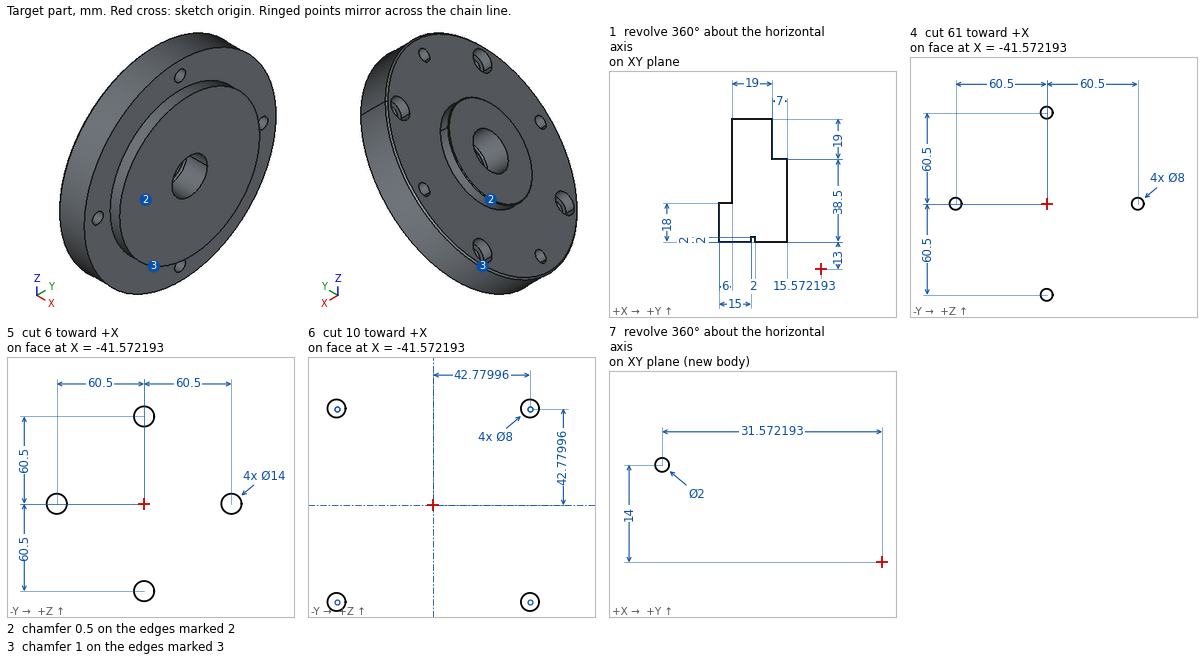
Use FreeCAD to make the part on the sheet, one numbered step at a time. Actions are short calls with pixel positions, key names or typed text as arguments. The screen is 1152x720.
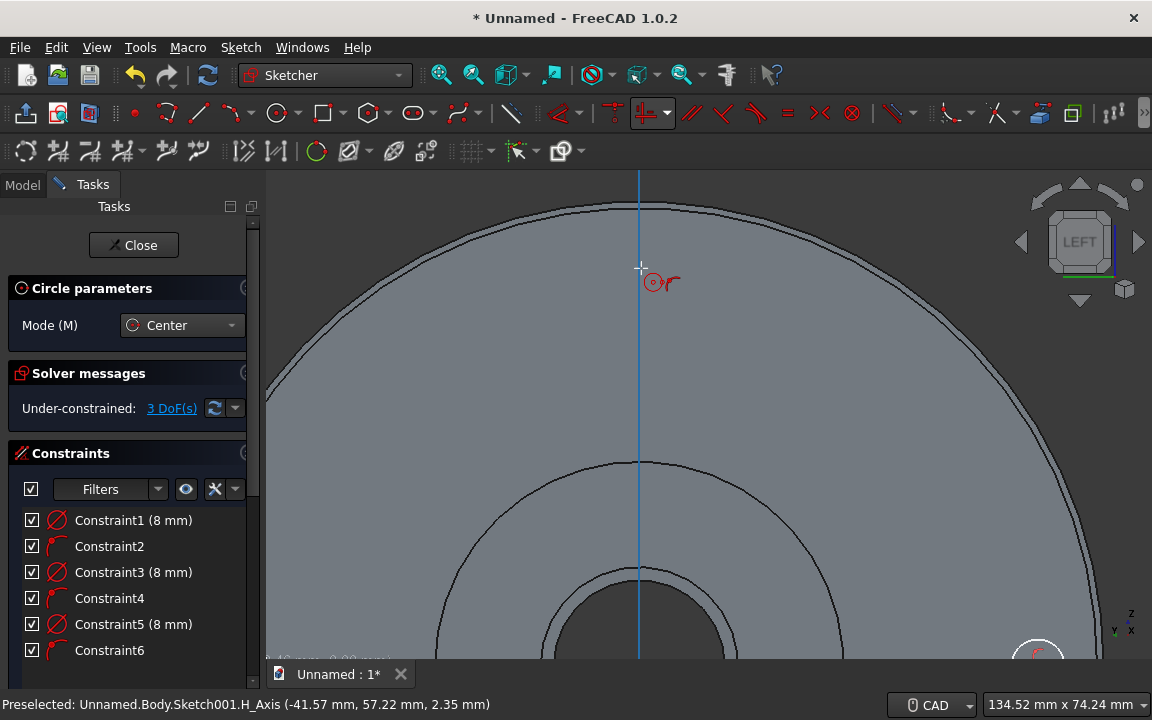
click(639, 267)
move(658, 249)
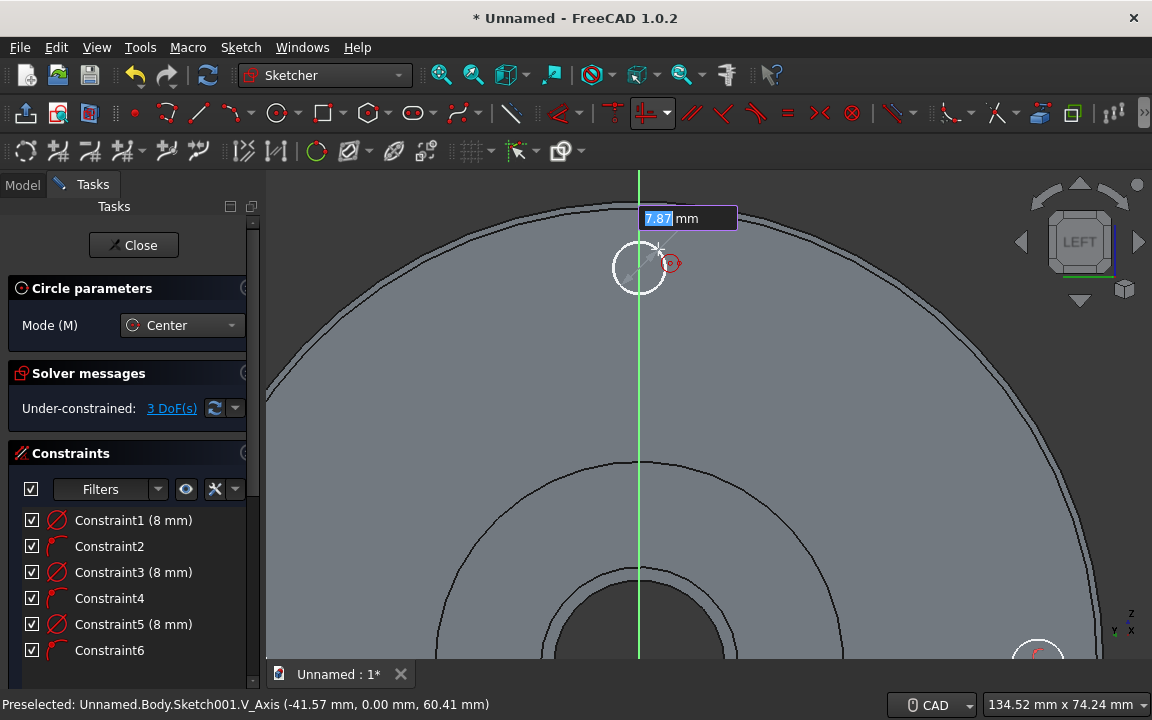
text(8)
key(Return)
key(Escape)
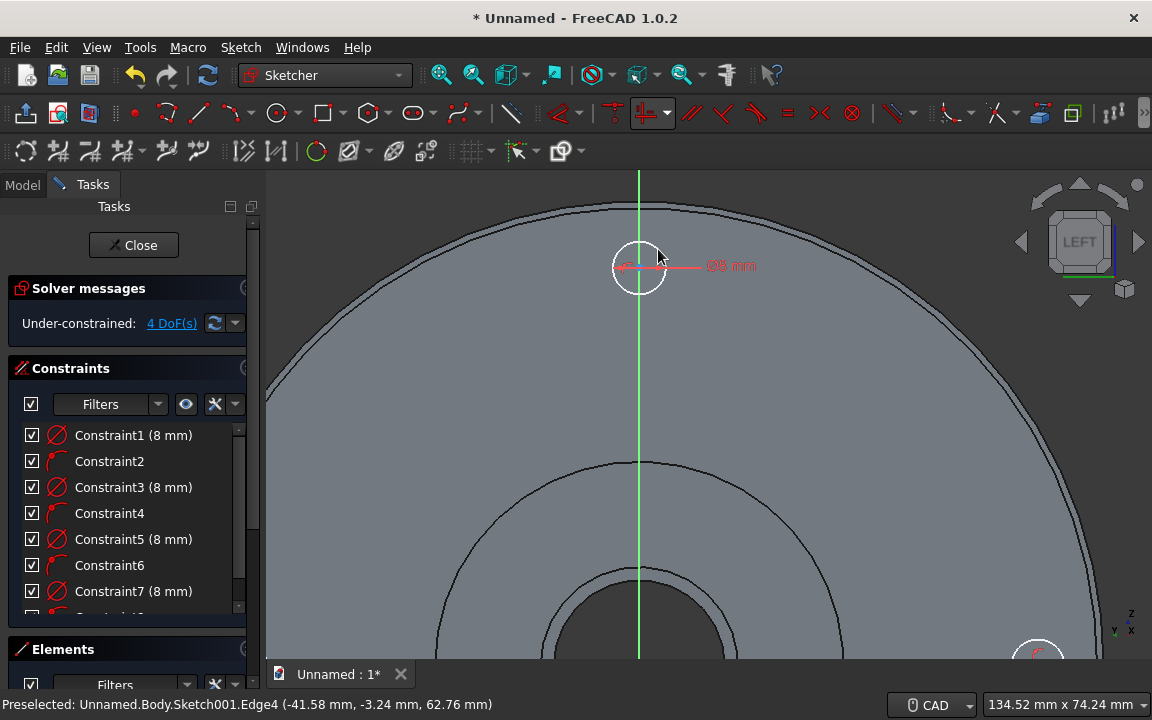
click(558, 114)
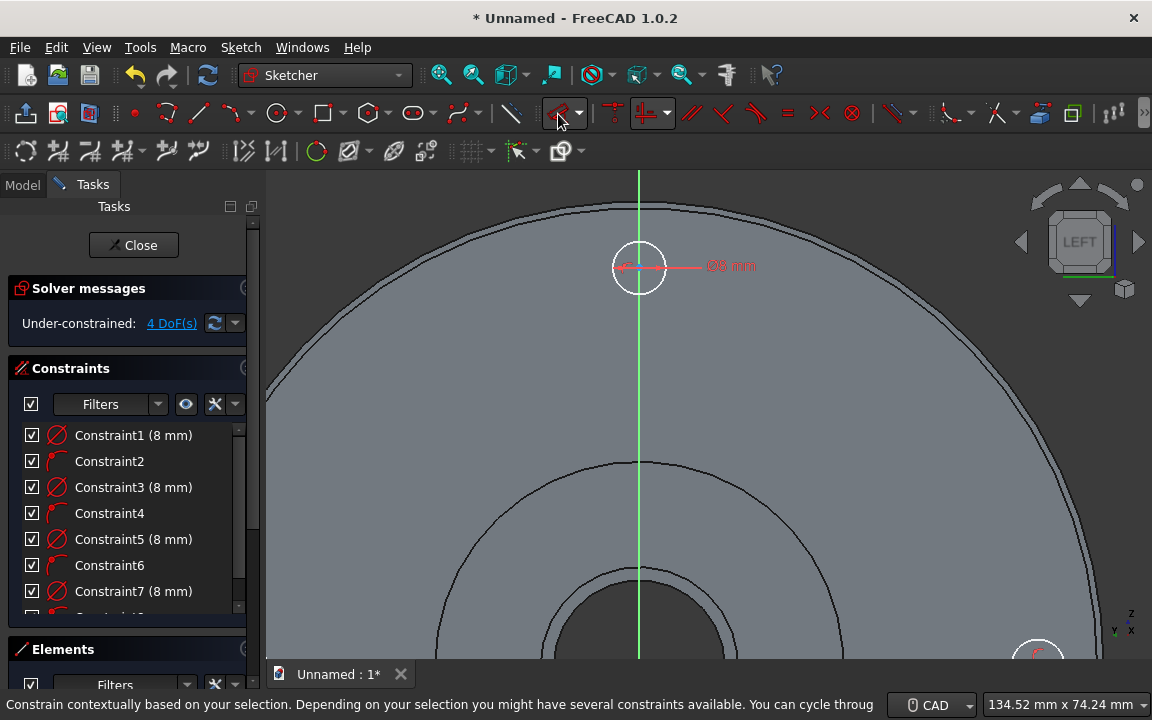
scroll(641, 268, down, 5)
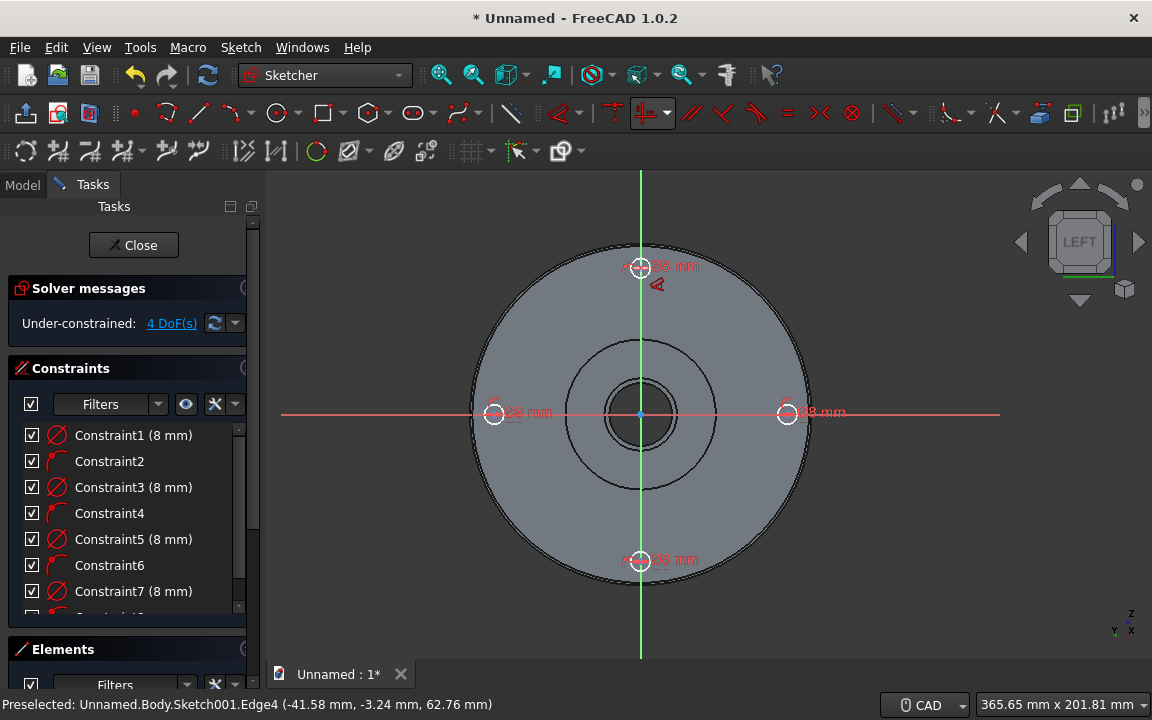
click(787, 415)
click(714, 449)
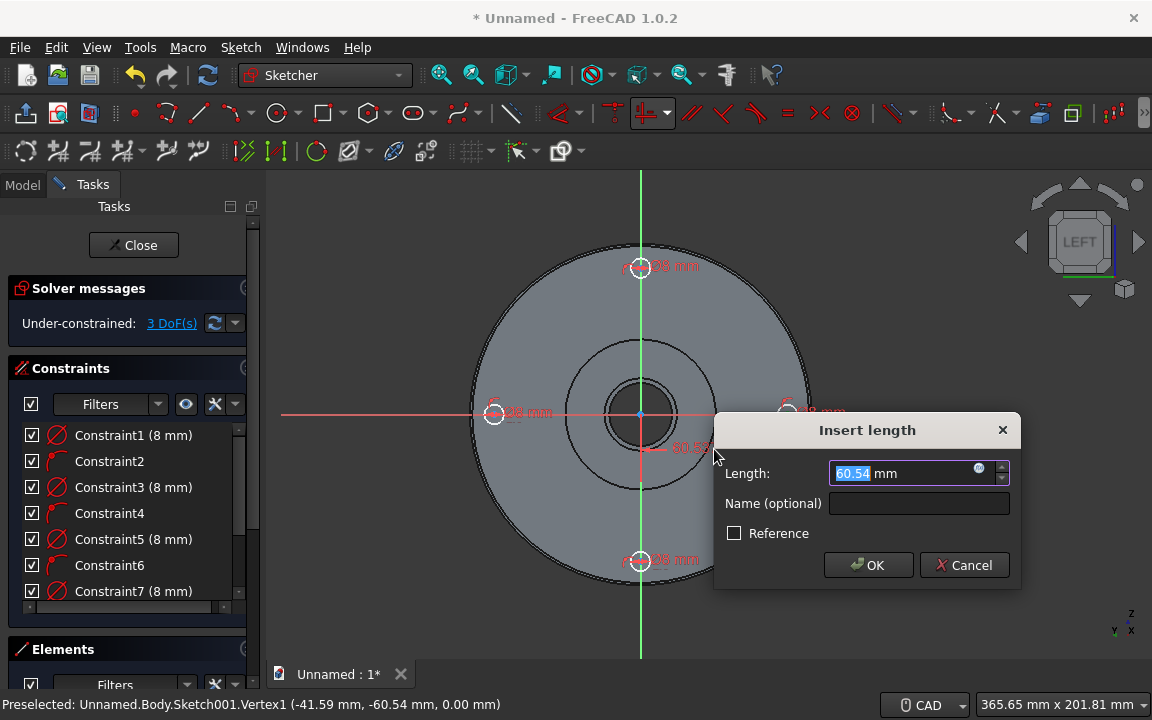
text(60.5)
key(Return)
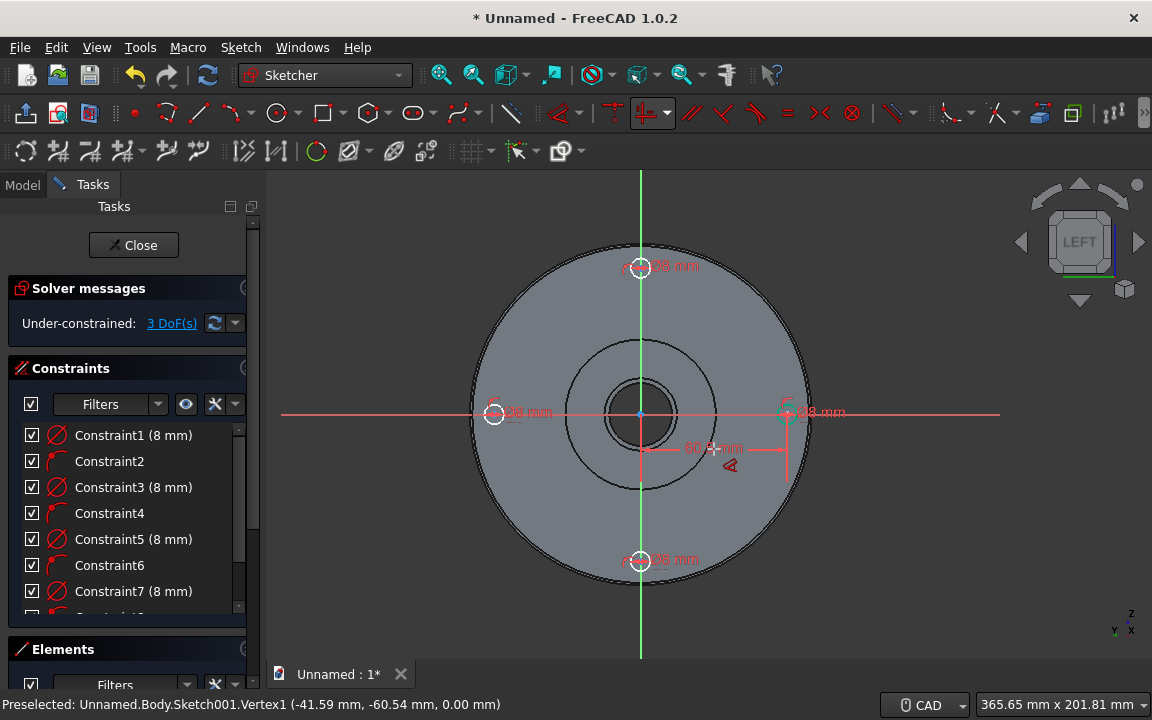
click(641, 562)
click(675, 488)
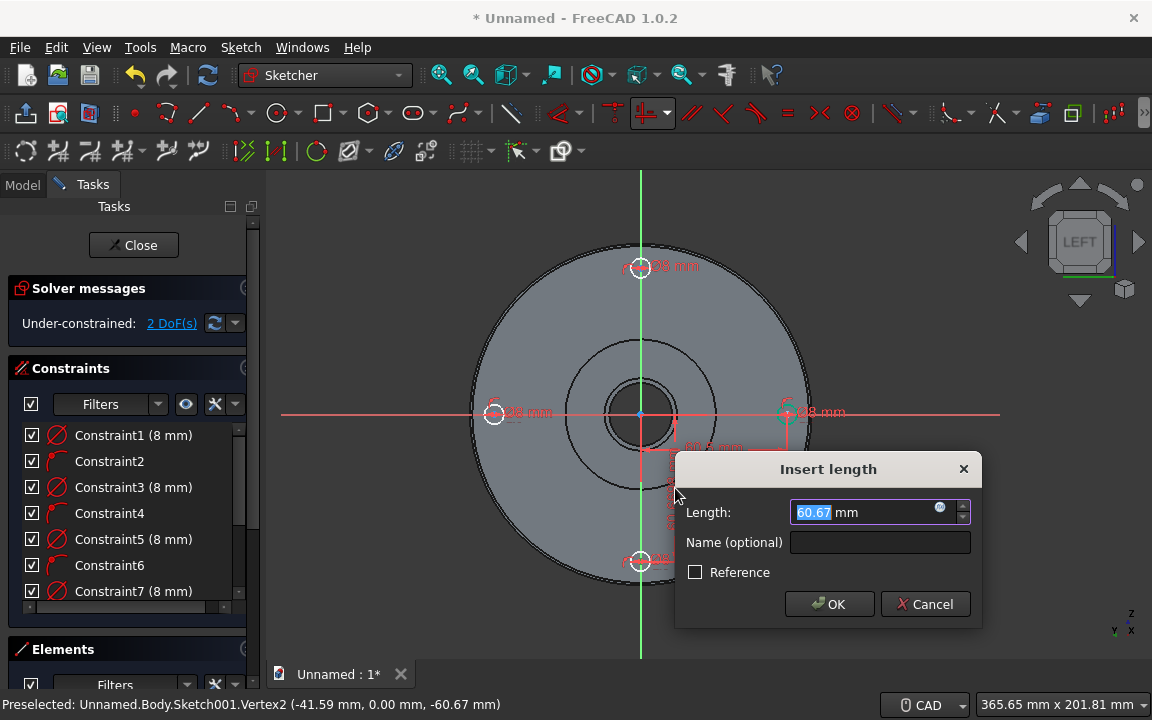
text(60.5)
key(Return)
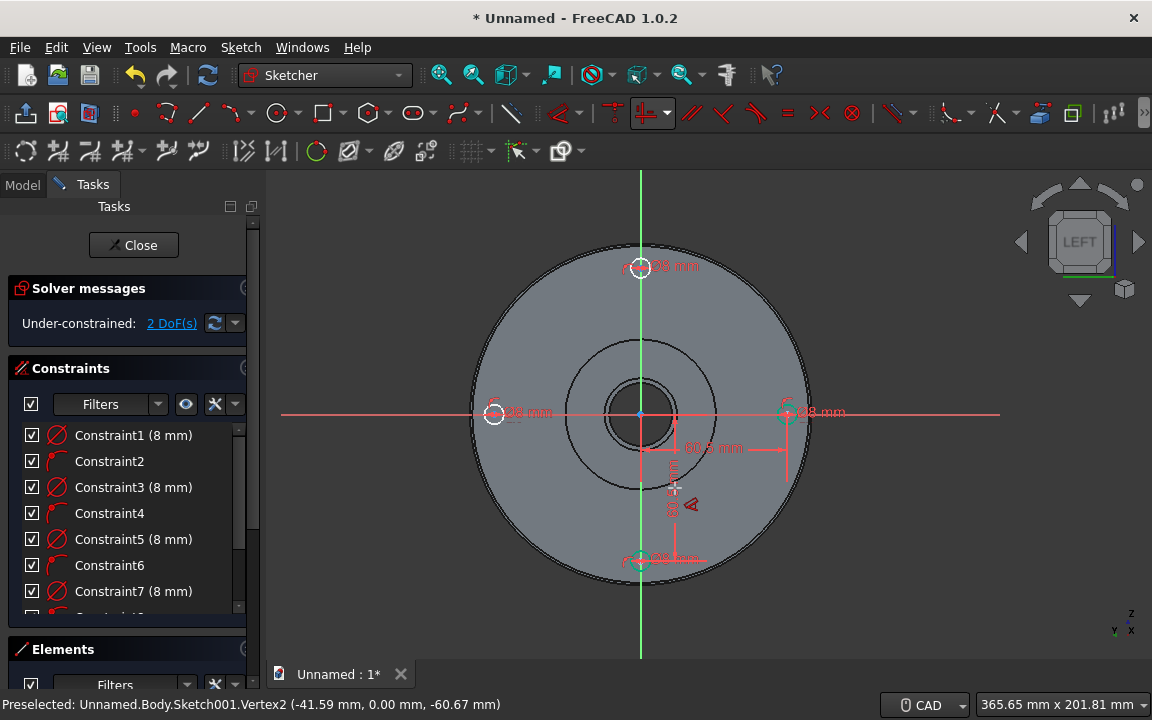
click(494, 415)
click(567, 449)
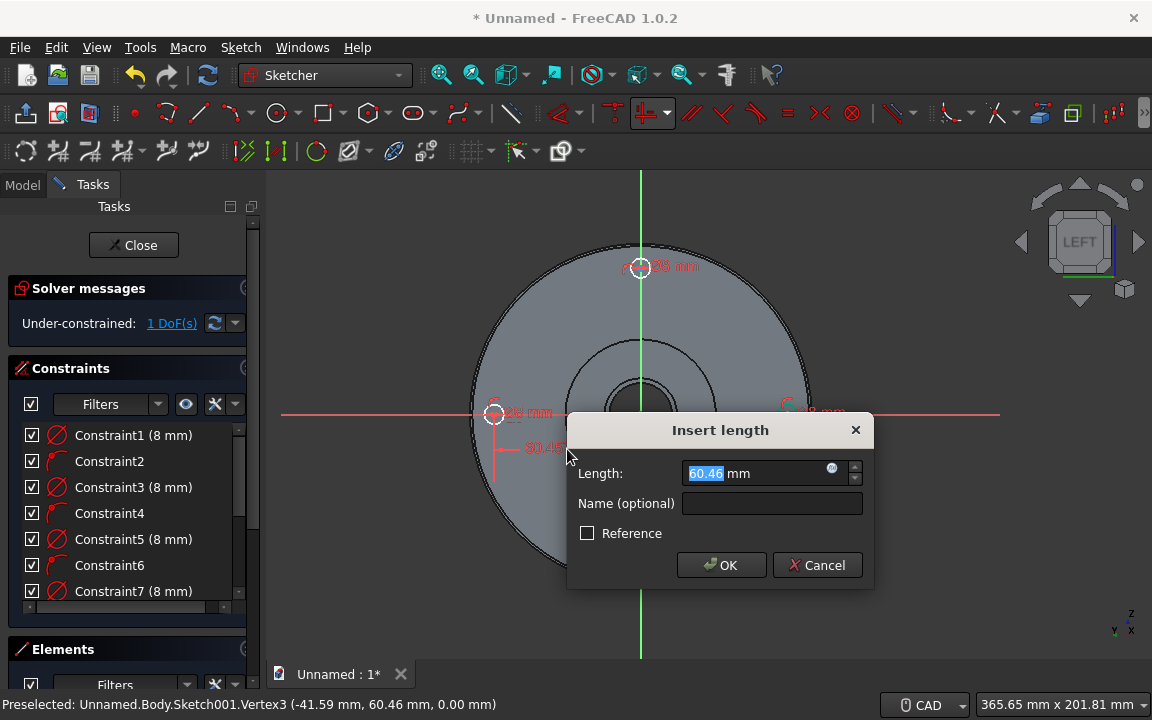
text(60.5)
key(Return)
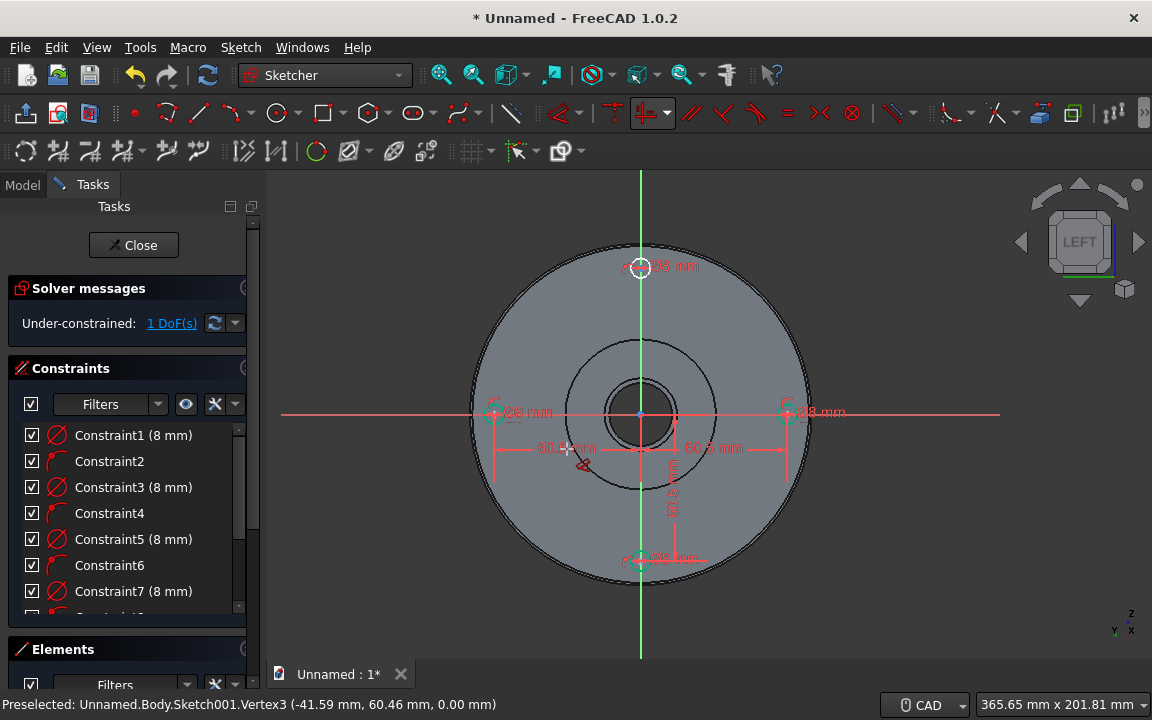
click(641, 268)
click(675, 341)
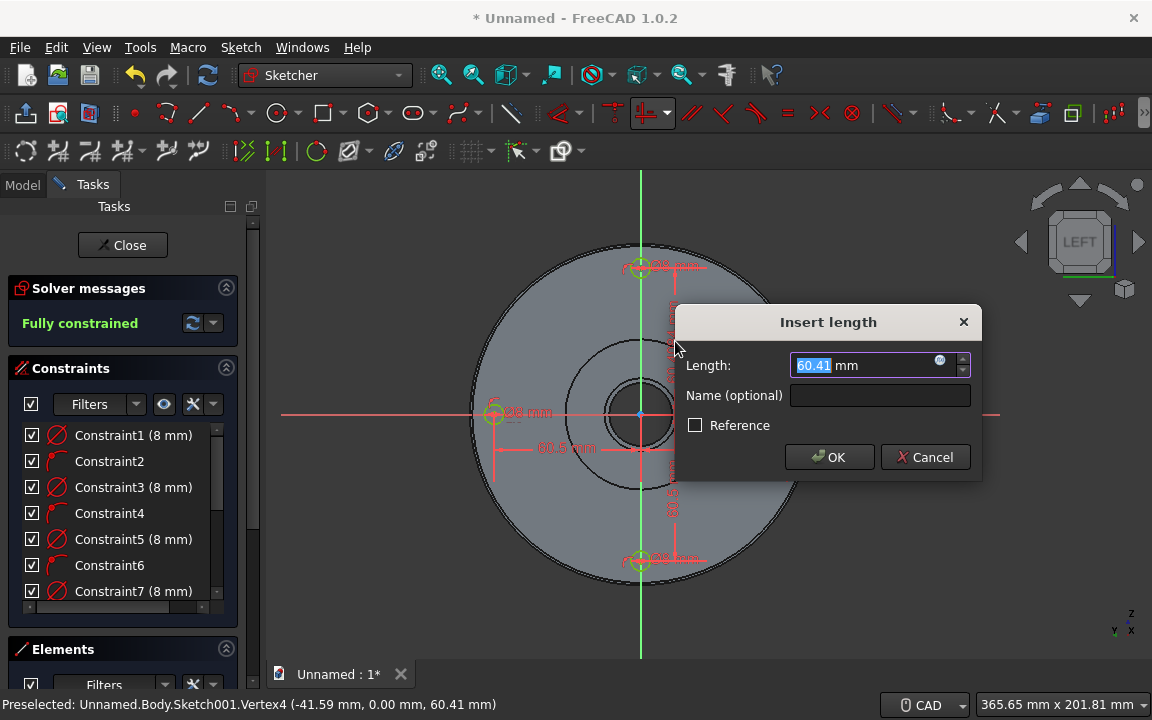
text(60.5)
key(Return)
key(Escape)